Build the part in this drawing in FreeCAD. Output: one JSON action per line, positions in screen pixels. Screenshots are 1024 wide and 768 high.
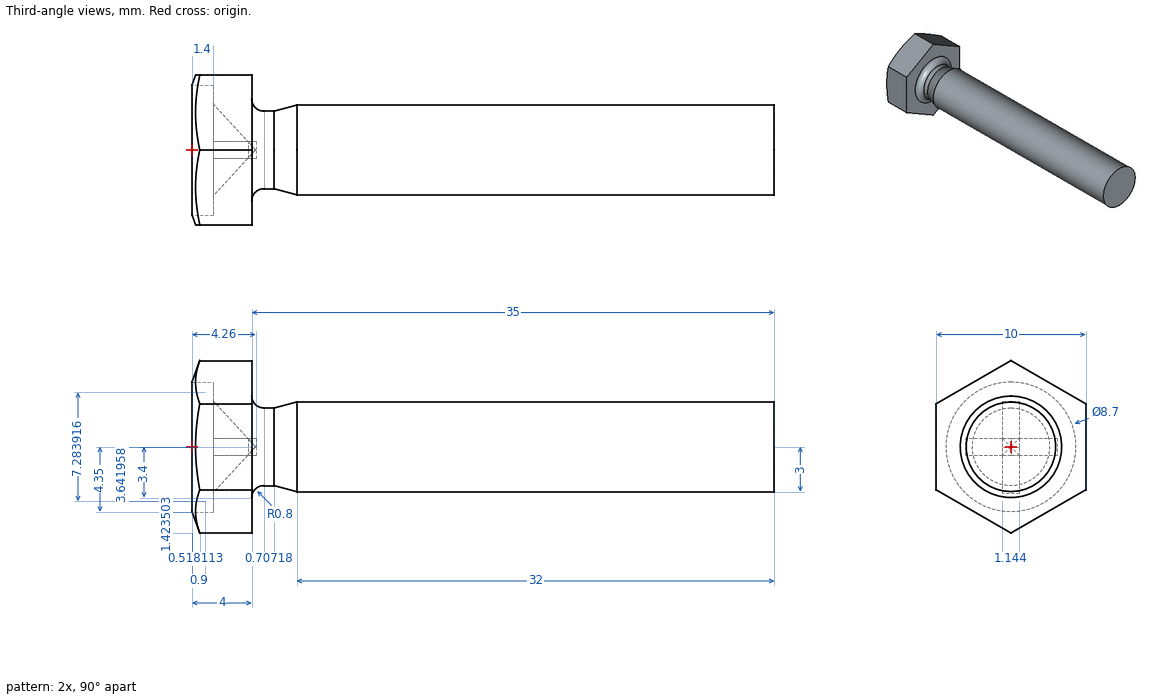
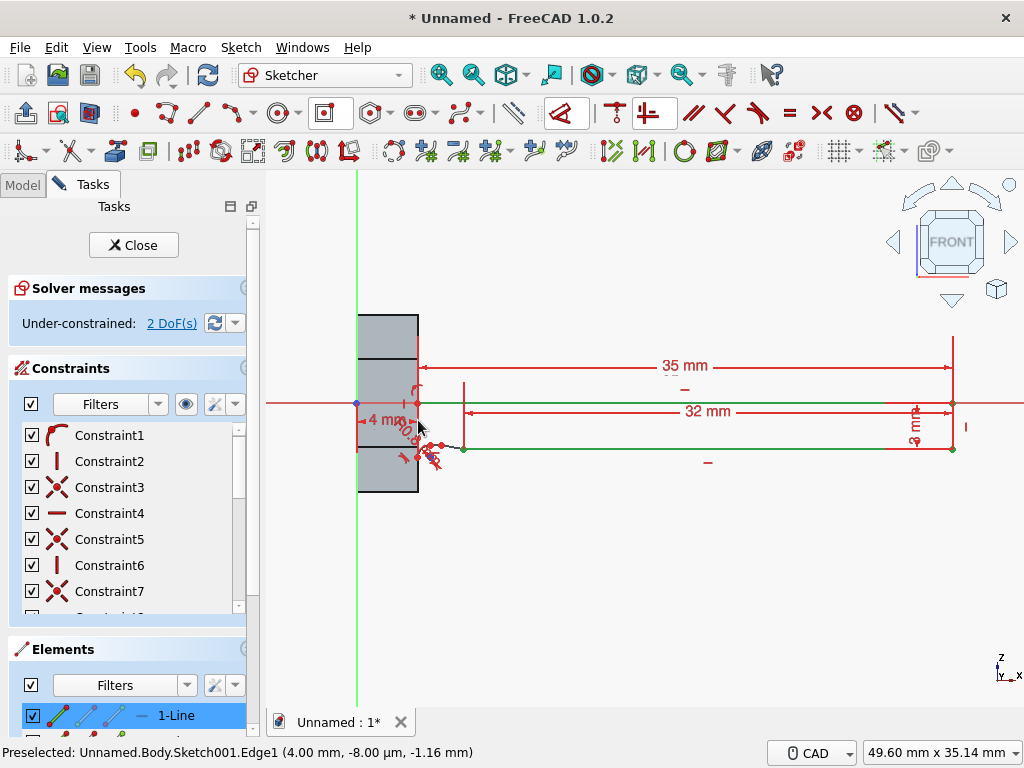
{"action": "left_click", "coordinate": [584, 114]}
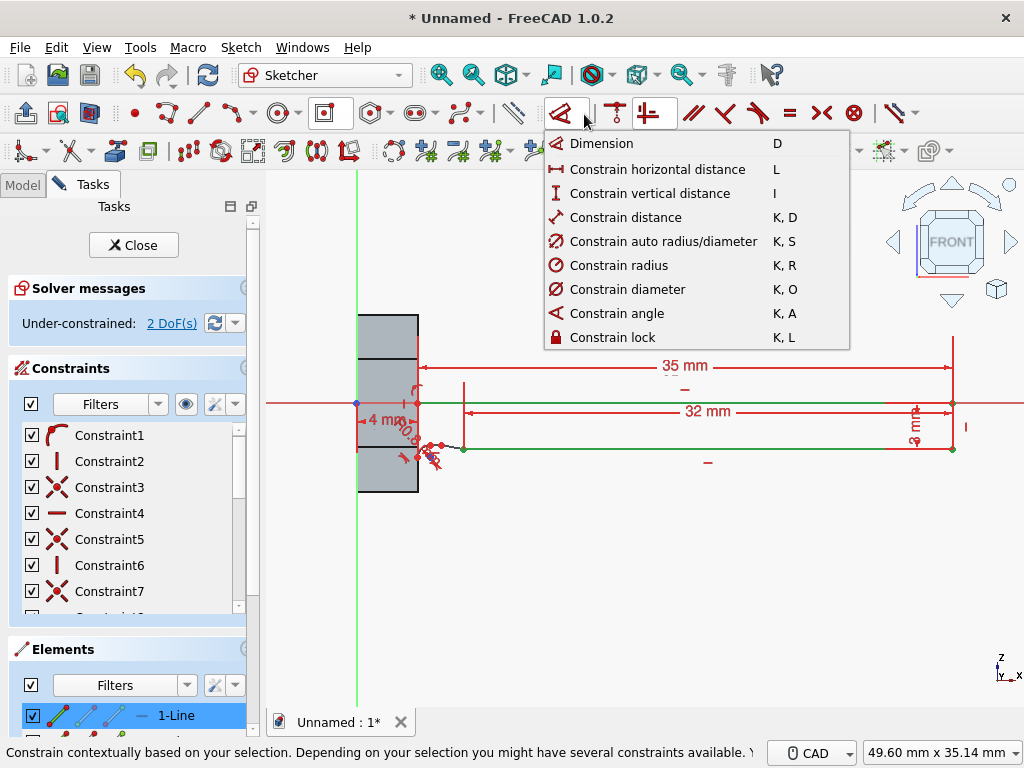
{"action": "left_click", "coordinate": [697, 193]}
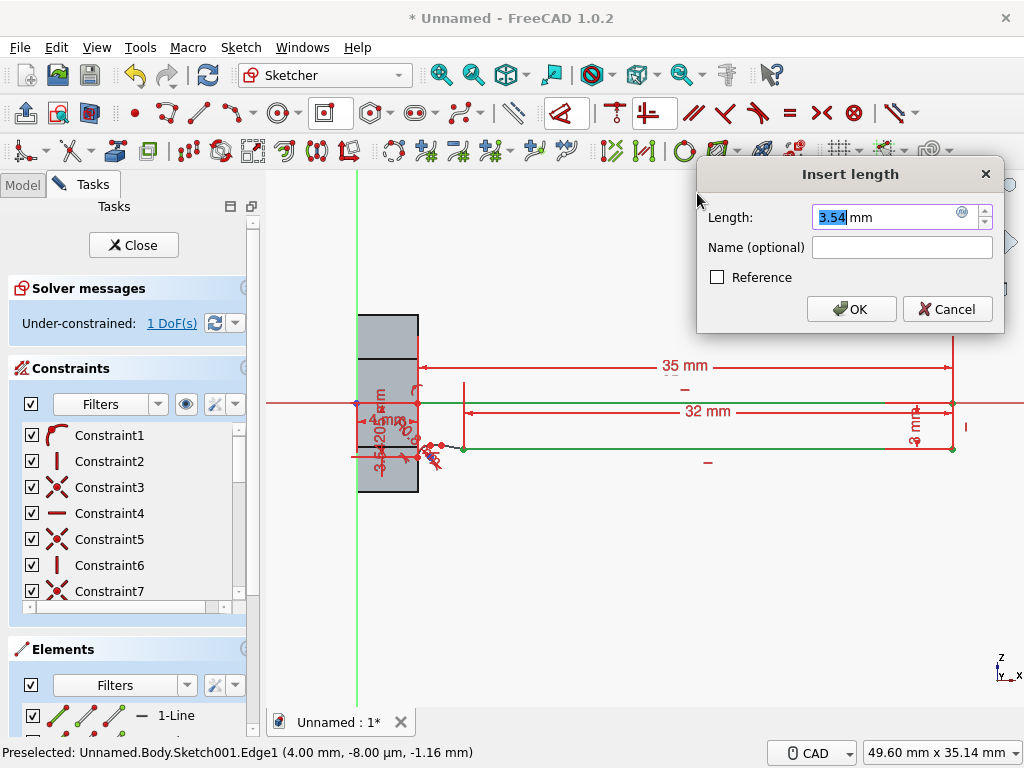
{"action": "type", "text": "3.4"}
{"action": "key", "text": "Return"}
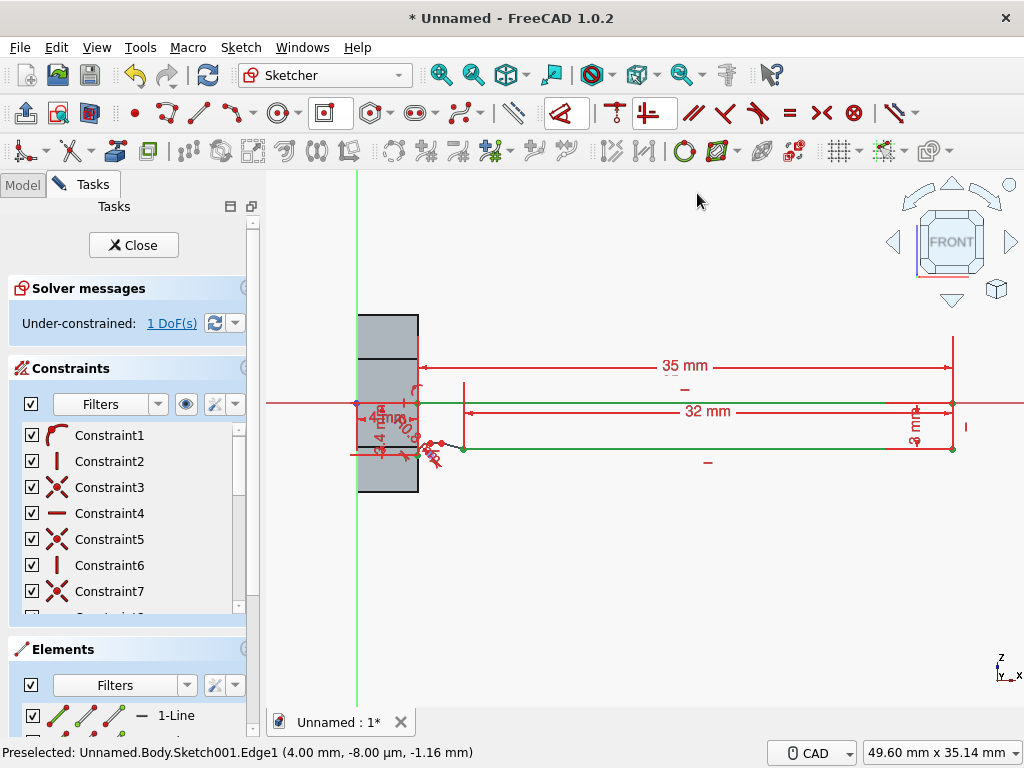
{"action": "scroll", "coordinate": [436, 443], "scroll_direction": "up", "scroll_amount": 7}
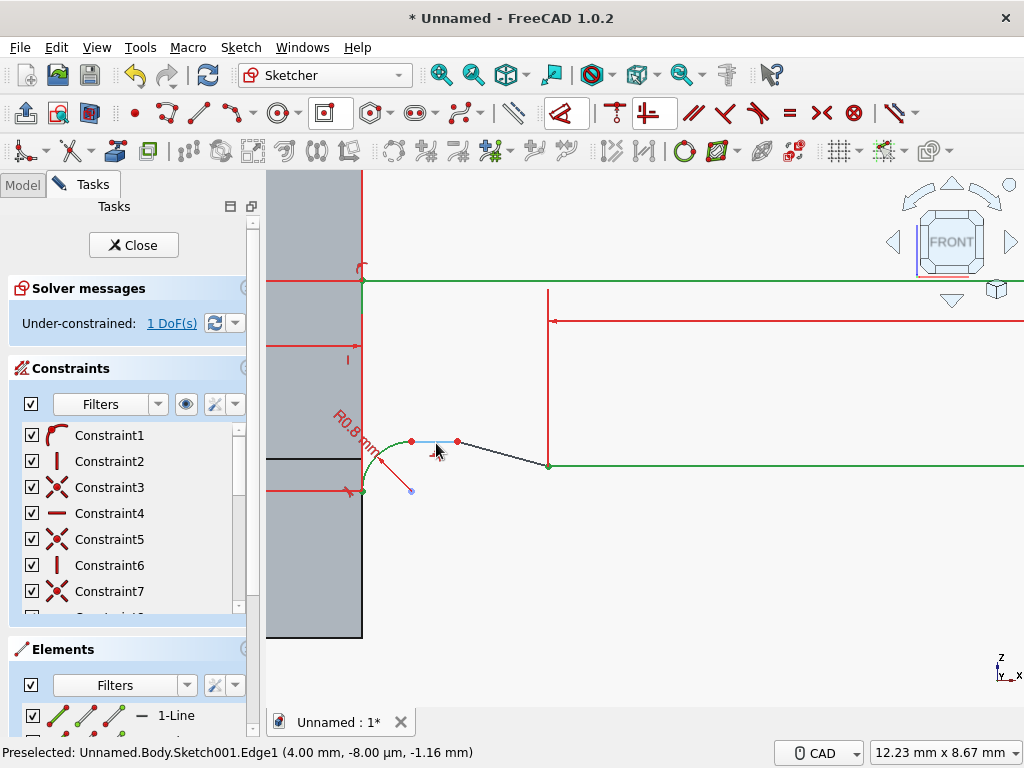
{"action": "left_click", "coordinate": [435, 442]}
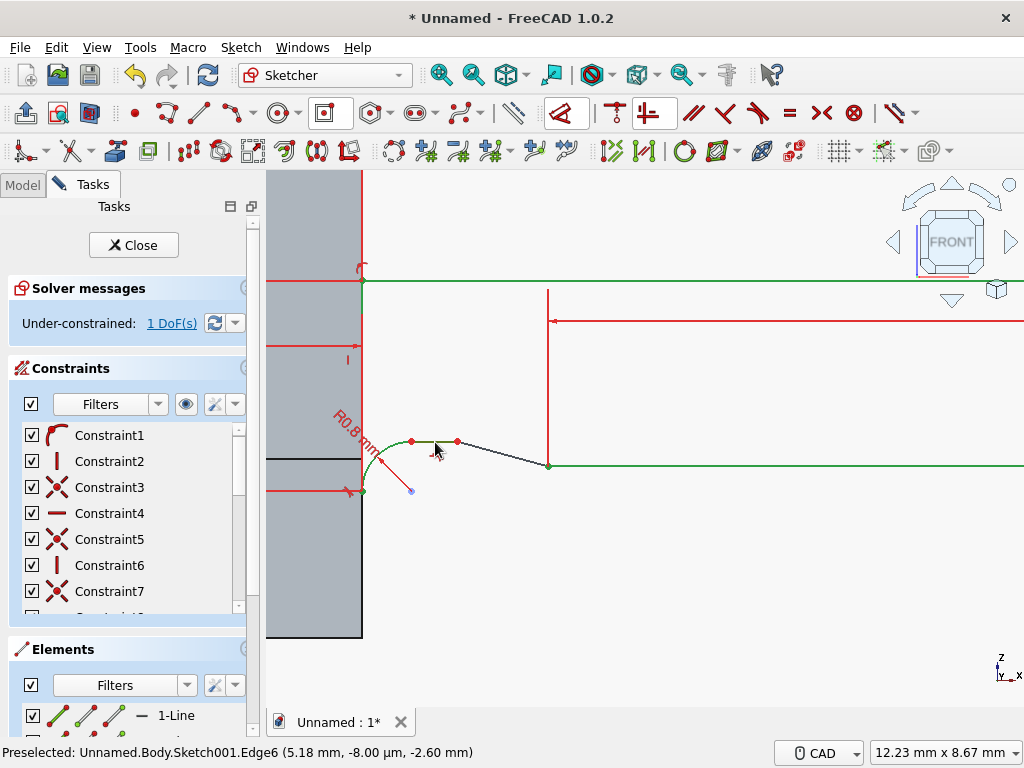
{"action": "key", "text": "l"}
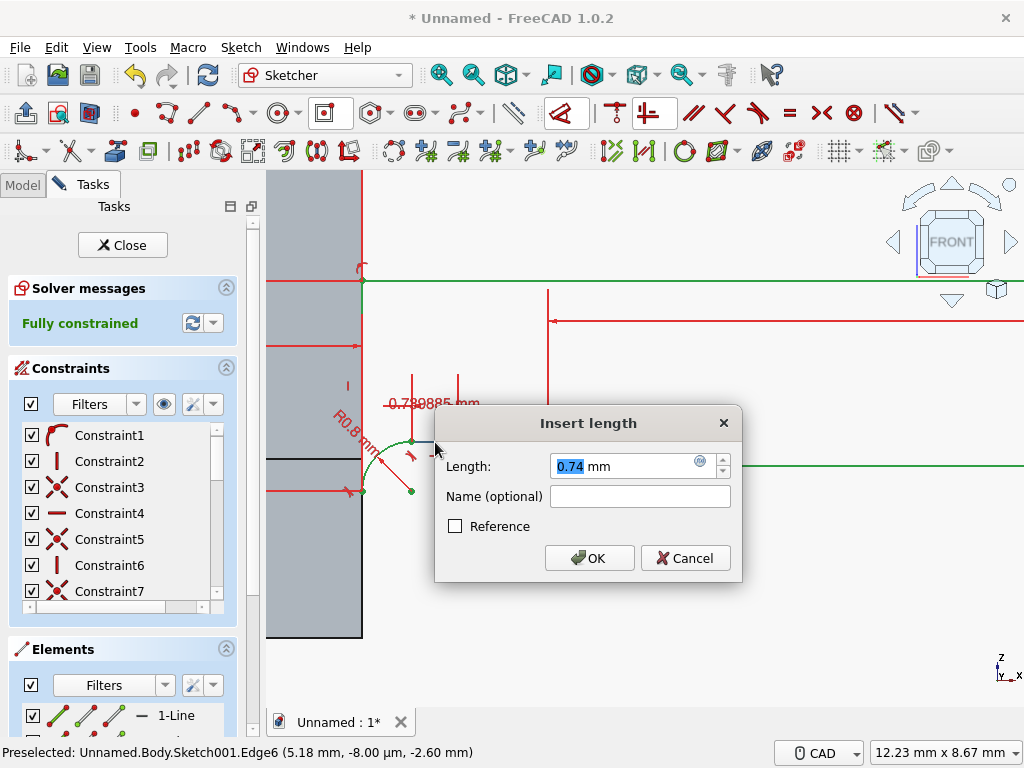
{"action": "type", "text": "0.70718"}
{"action": "key", "text": "Return"}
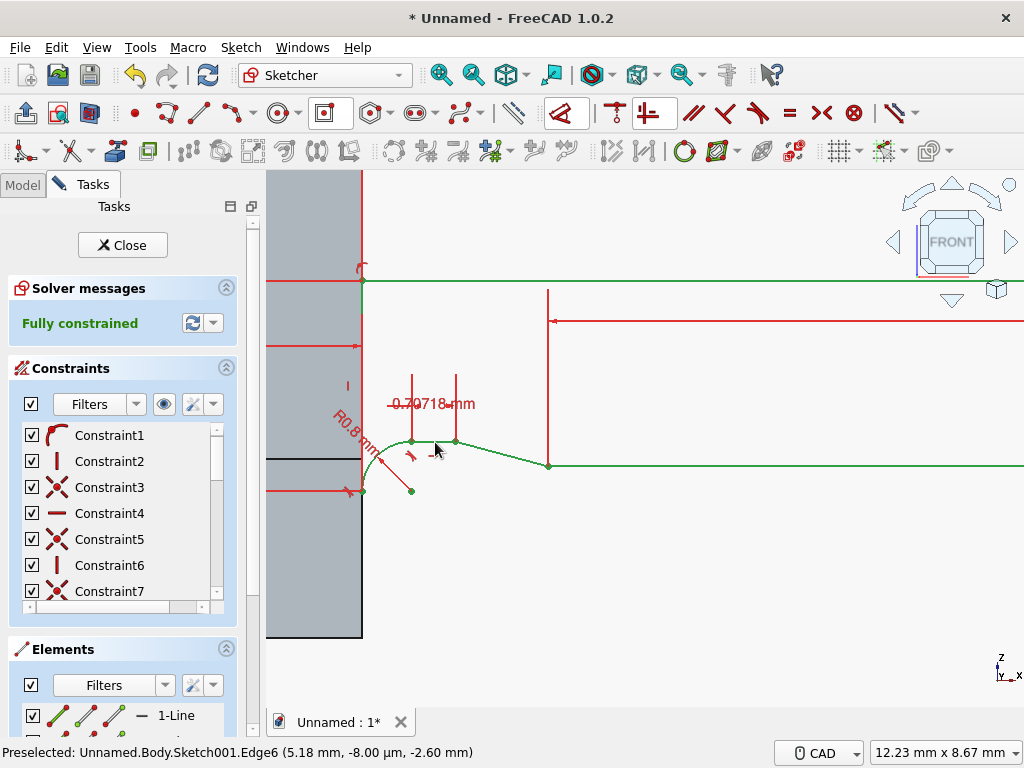
{"action": "left_click", "coordinate": [123, 245]}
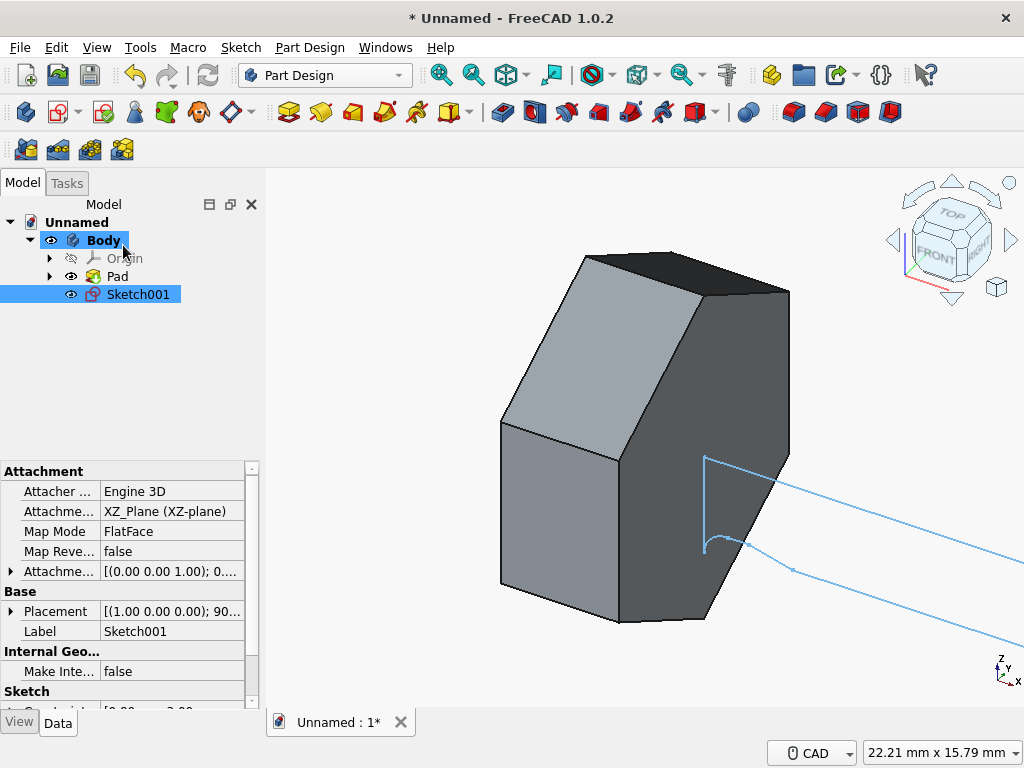
{"action": "left_click", "coordinate": [322, 112]}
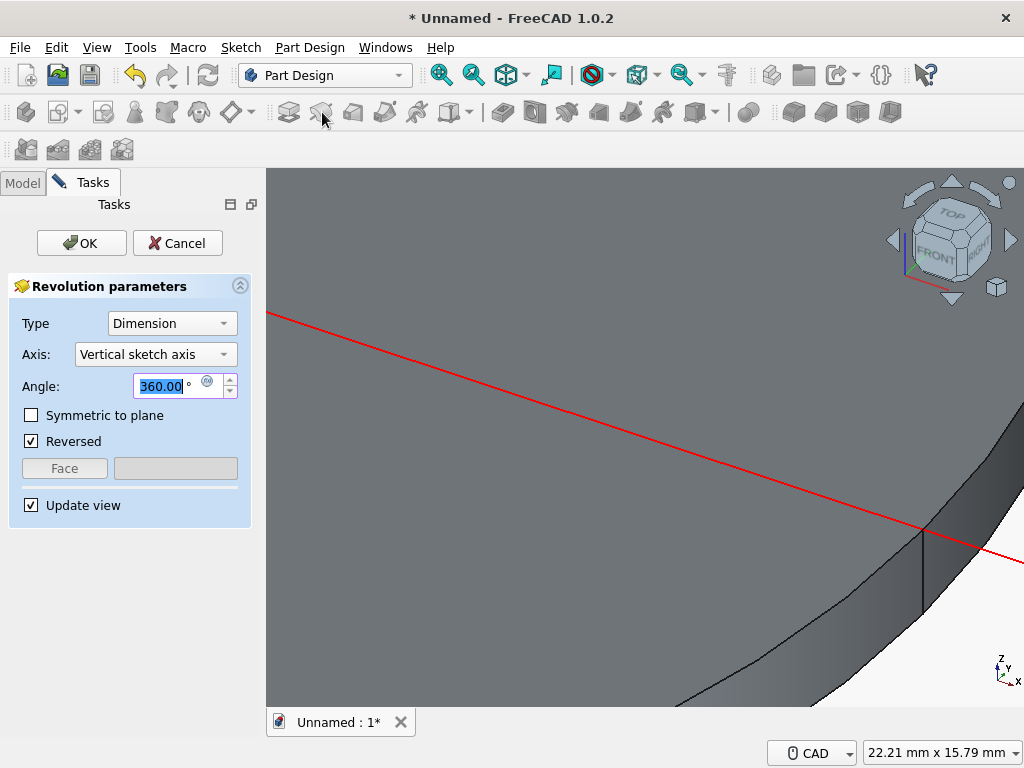
{"action": "left_click", "coordinate": [156, 354]}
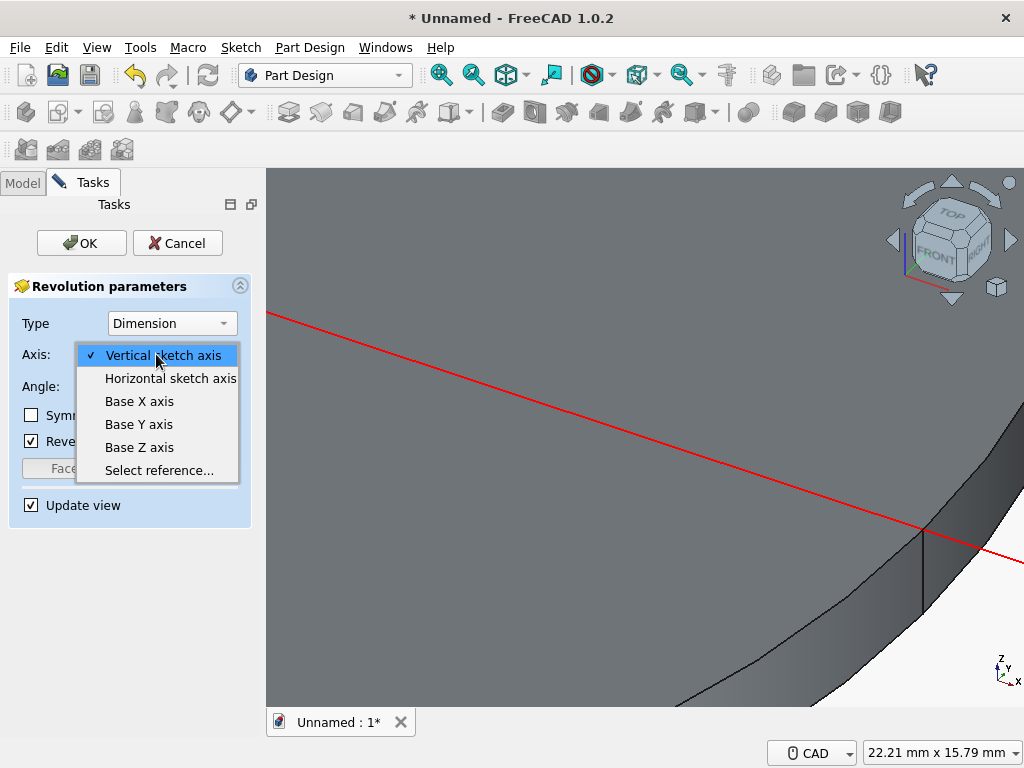
{"action": "left_click", "coordinate": [156, 378]}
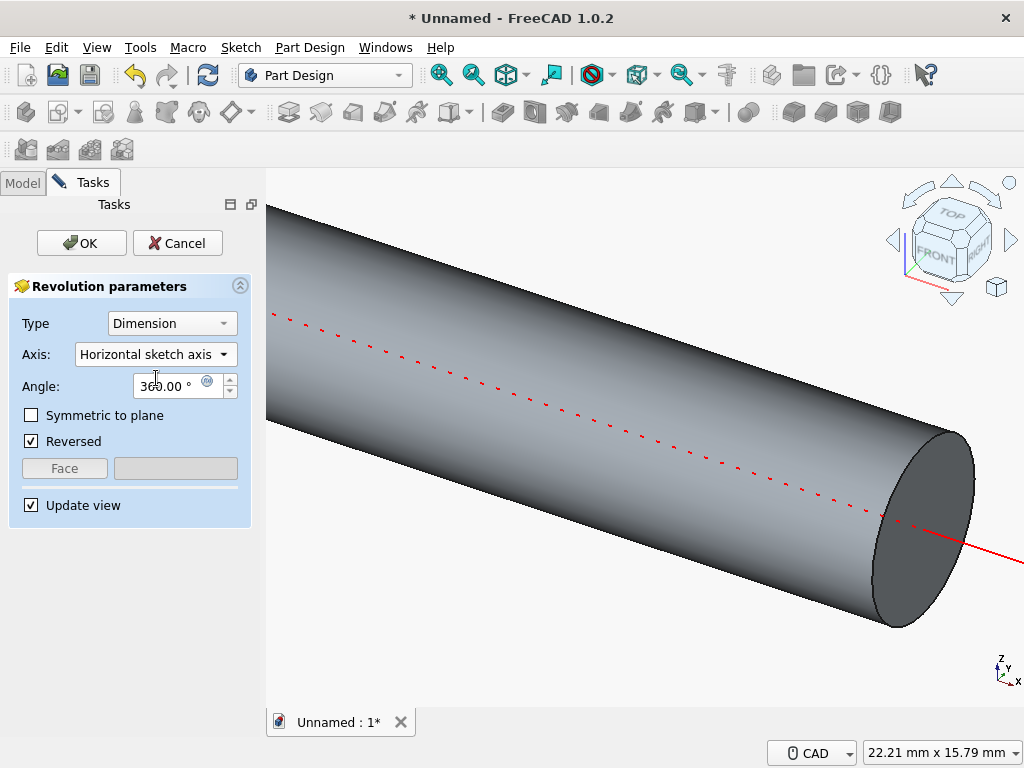
{"action": "left_click", "coordinate": [82, 243]}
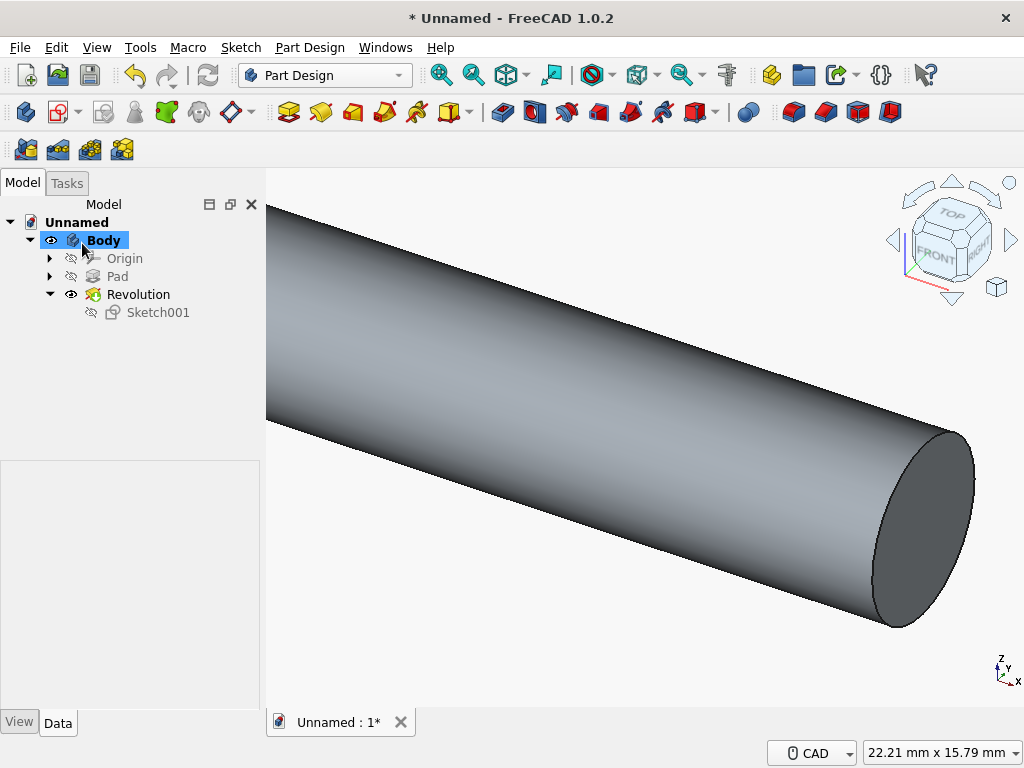
{"action": "key", "text": "v f"}